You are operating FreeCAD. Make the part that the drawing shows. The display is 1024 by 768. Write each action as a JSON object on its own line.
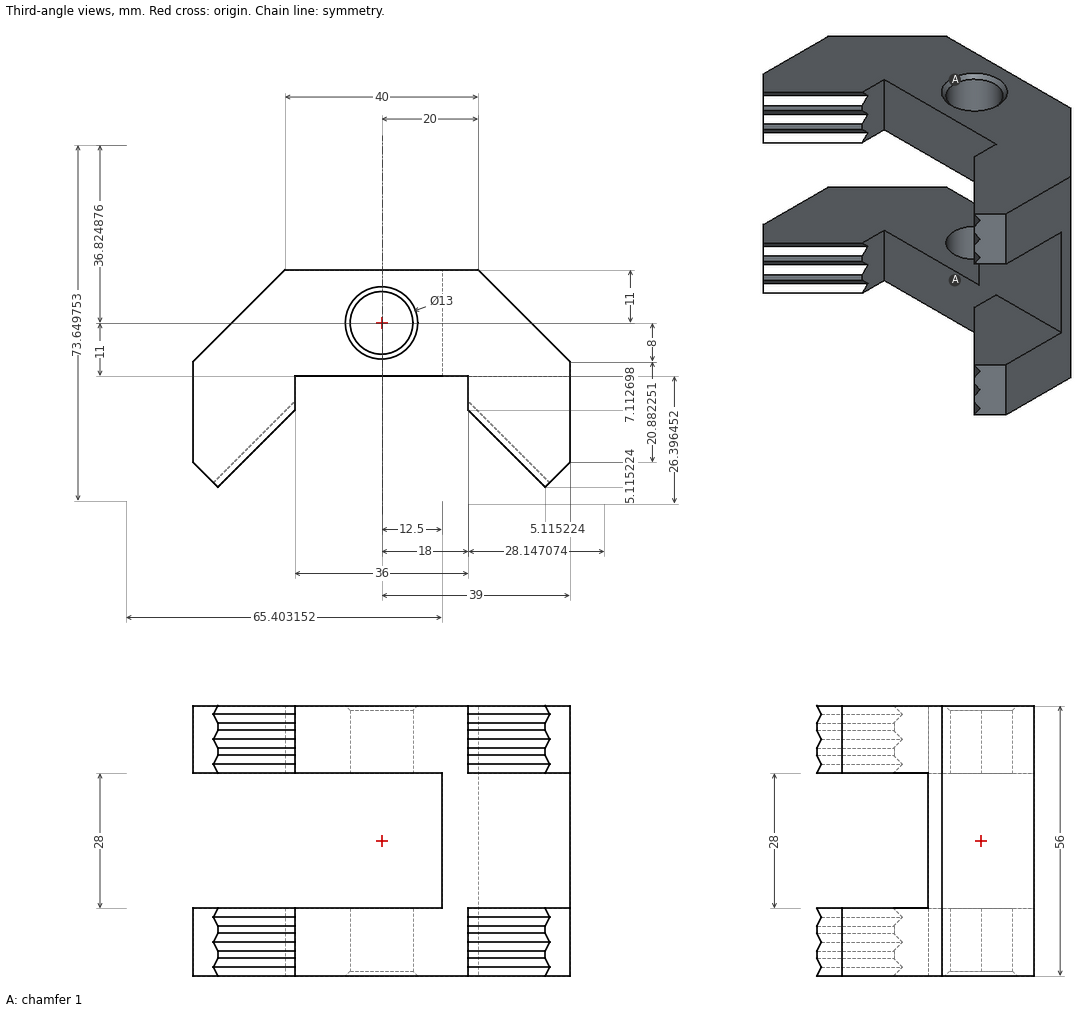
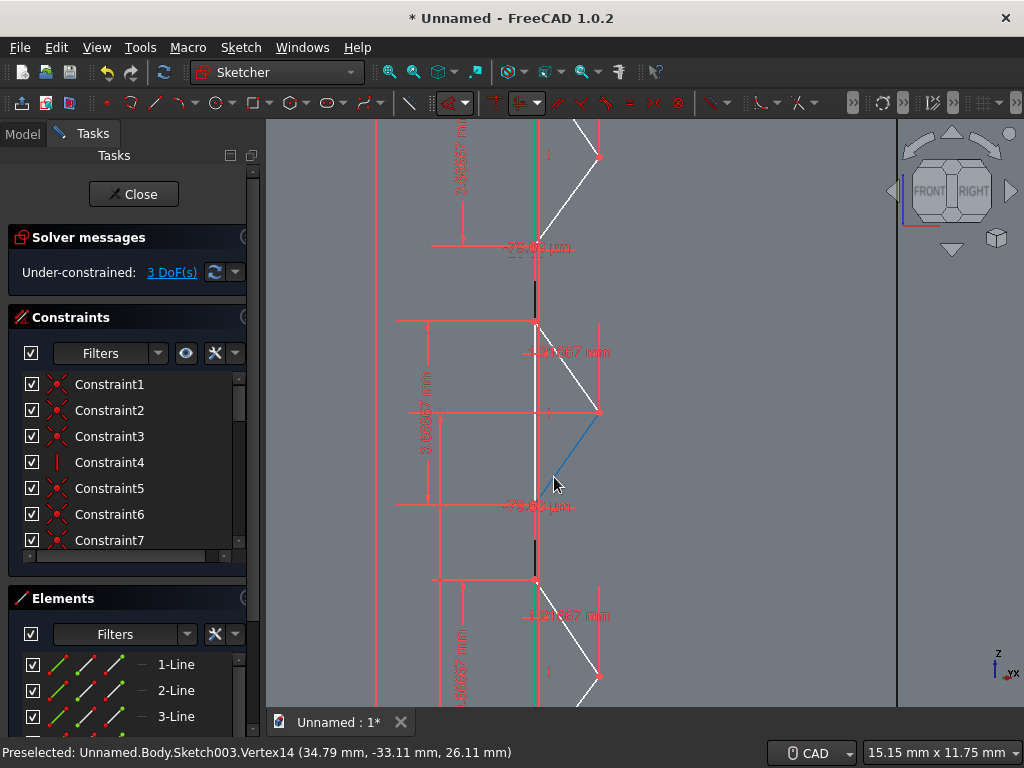
{"action": "left_click", "coordinate": [554, 477]}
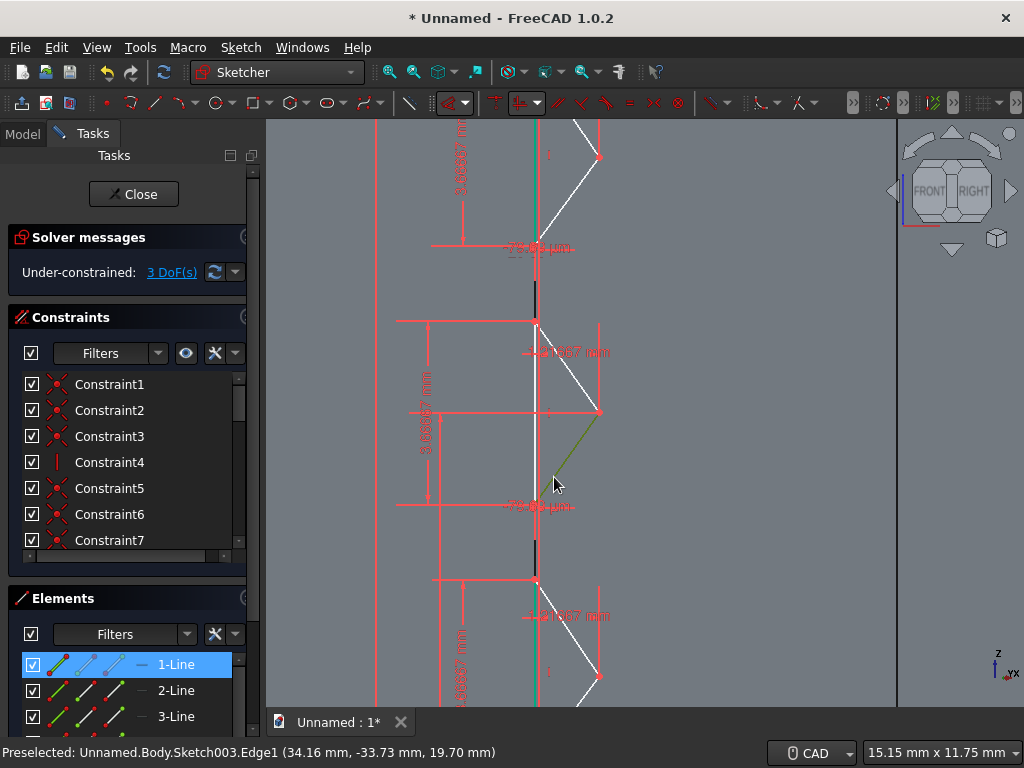
{"action": "key", "text": "i"}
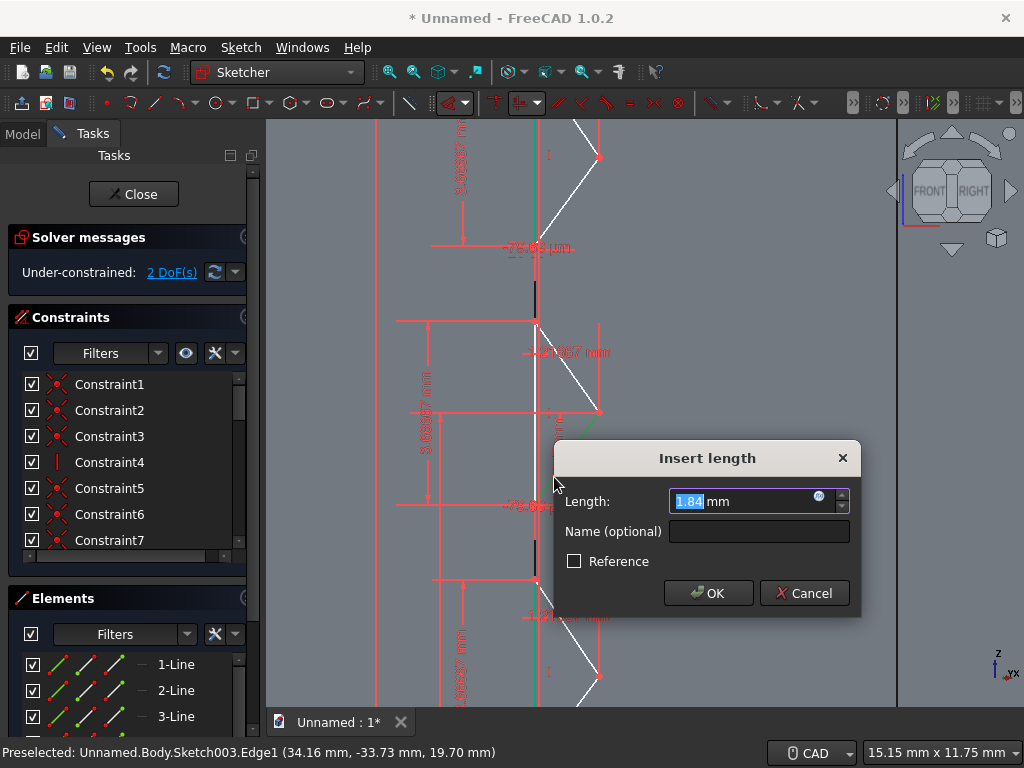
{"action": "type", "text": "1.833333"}
{"action": "key", "text": "Return"}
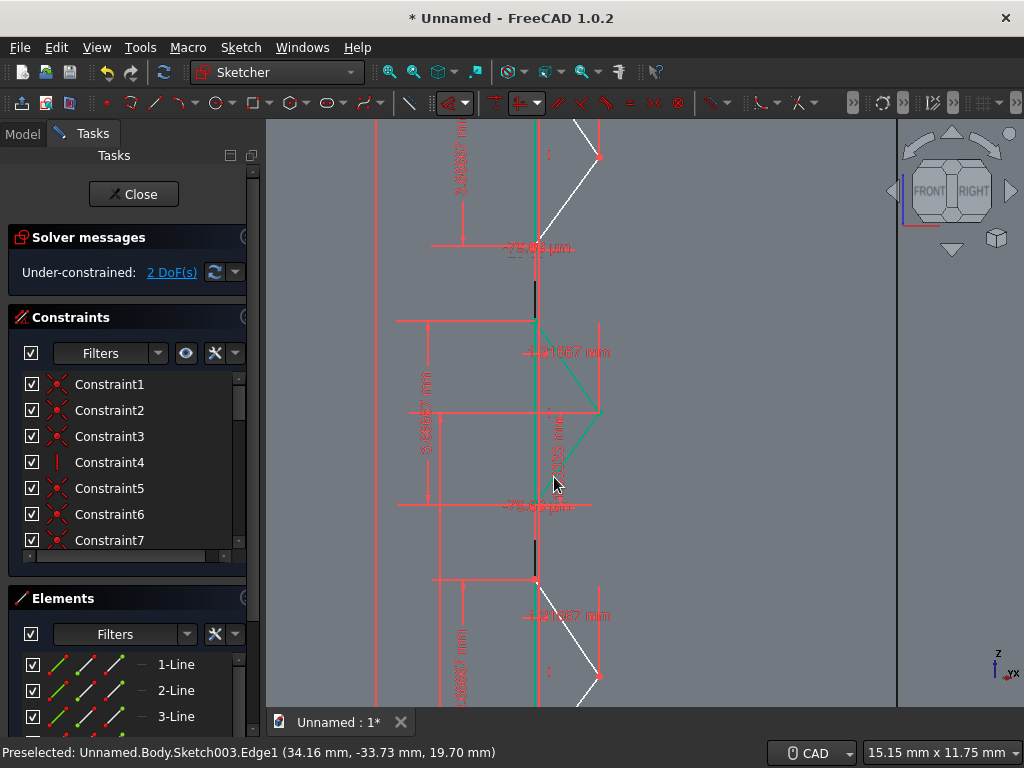
{"action": "scroll", "coordinate": [580, 298], "scroll_direction": "down", "scroll_amount": 7}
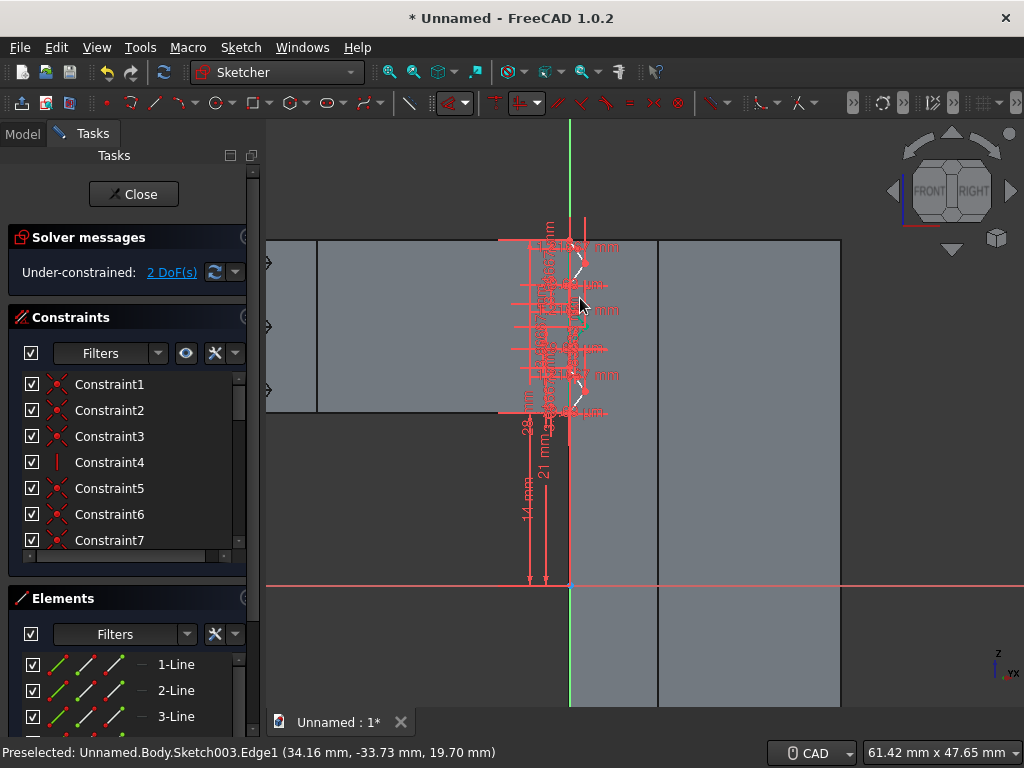
{"action": "scroll", "coordinate": [574, 406], "scroll_direction": "up", "scroll_amount": 7}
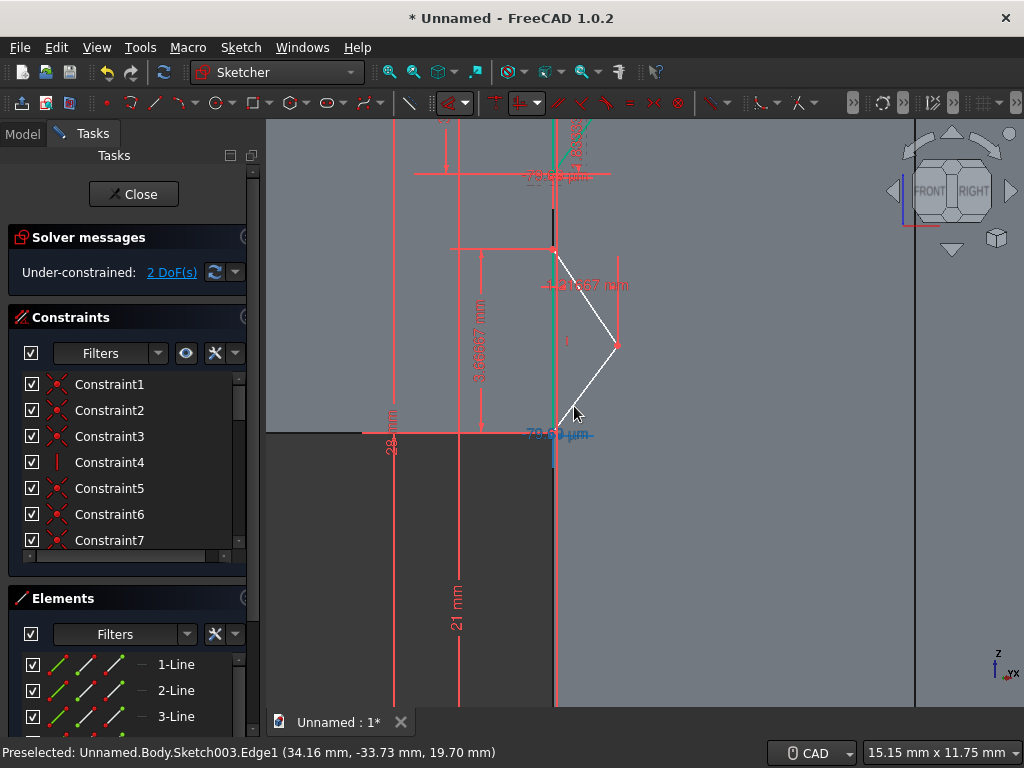
{"action": "left_click", "coordinate": [572, 407]}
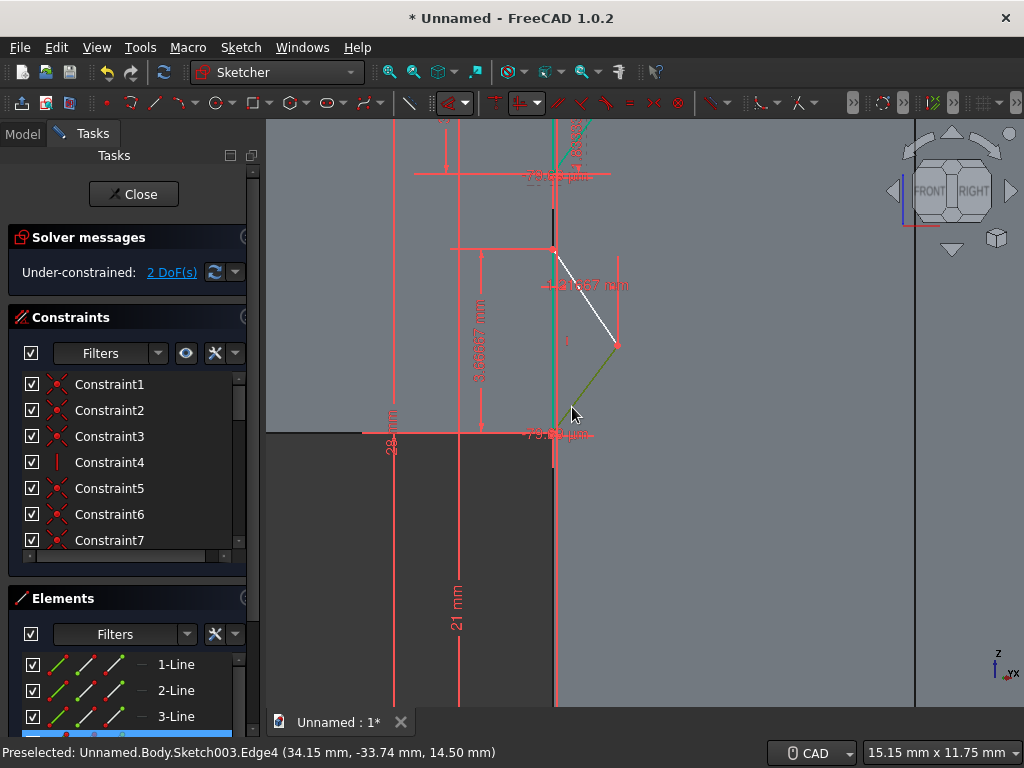
{"action": "left_click", "coordinate": [468, 104]}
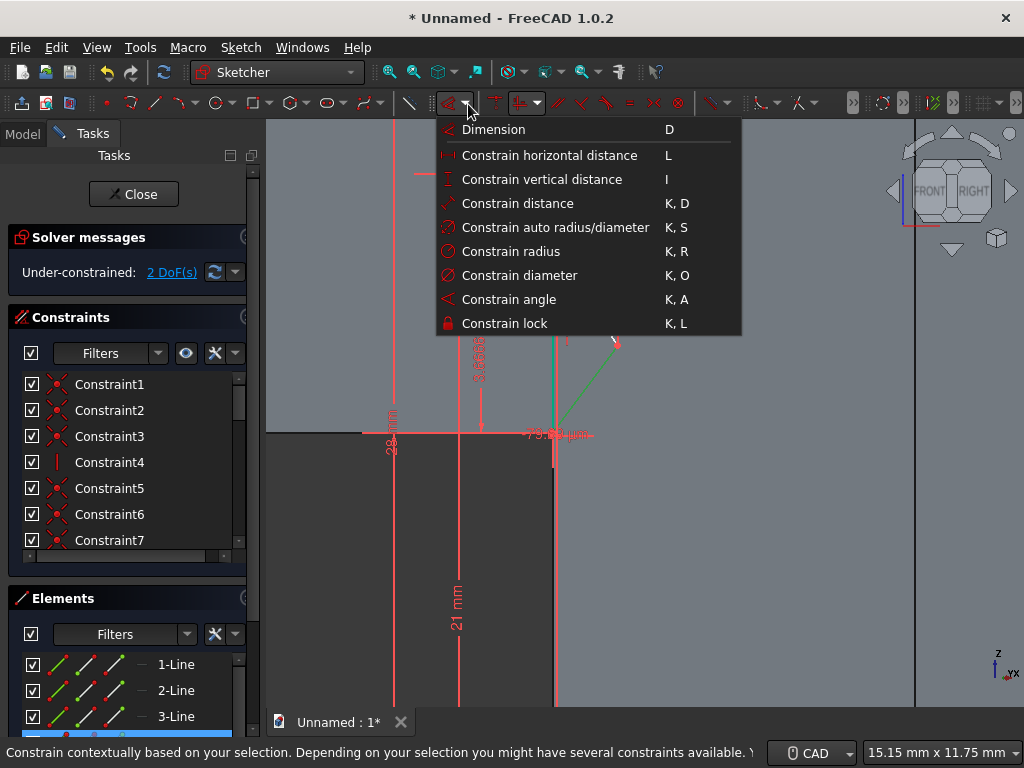
{"action": "left_click", "coordinate": [589, 179]}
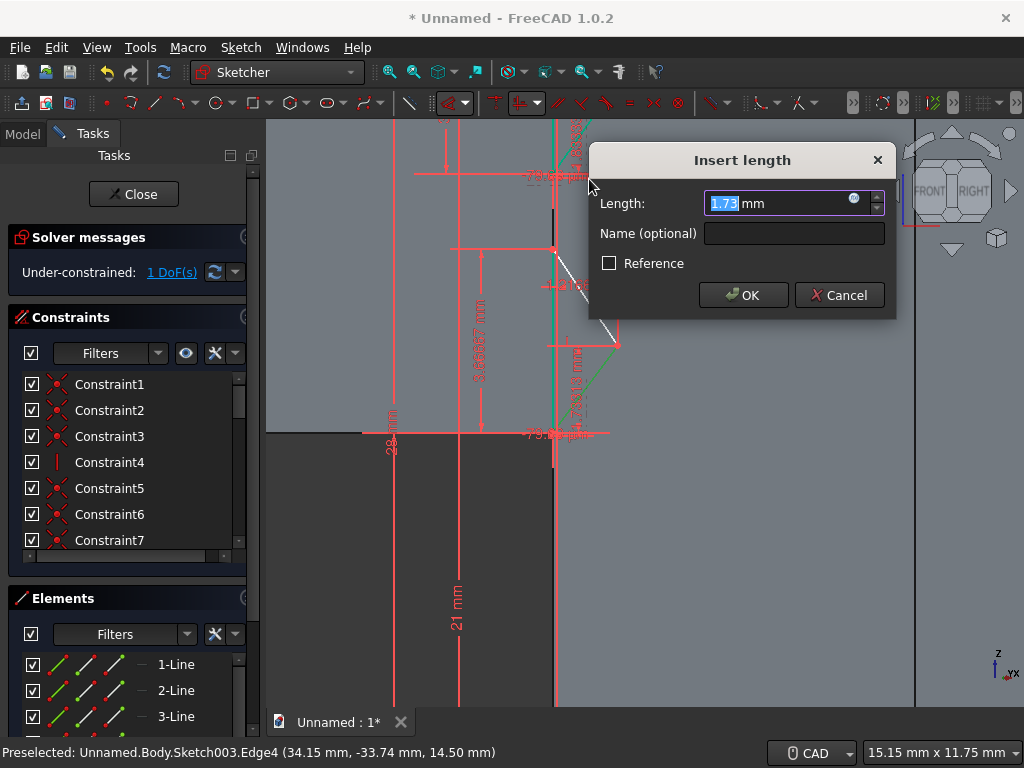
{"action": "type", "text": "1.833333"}
{"action": "key", "text": "Return"}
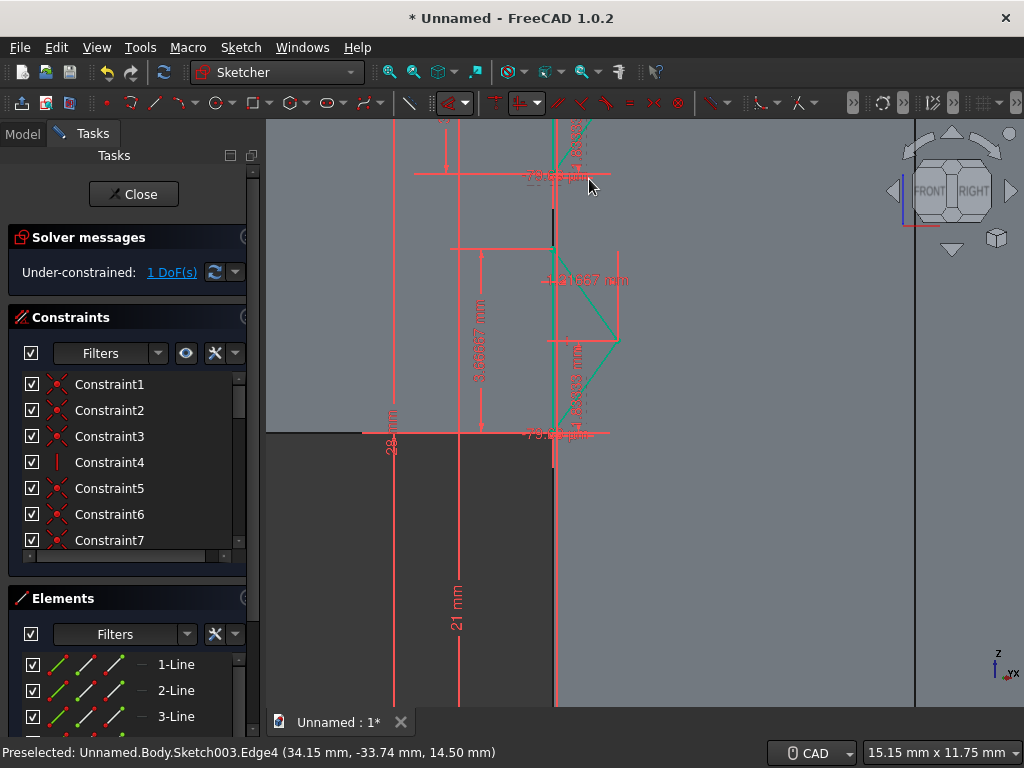
{"action": "scroll", "coordinate": [574, 407], "scroll_direction": "down", "scroll_amount": 7}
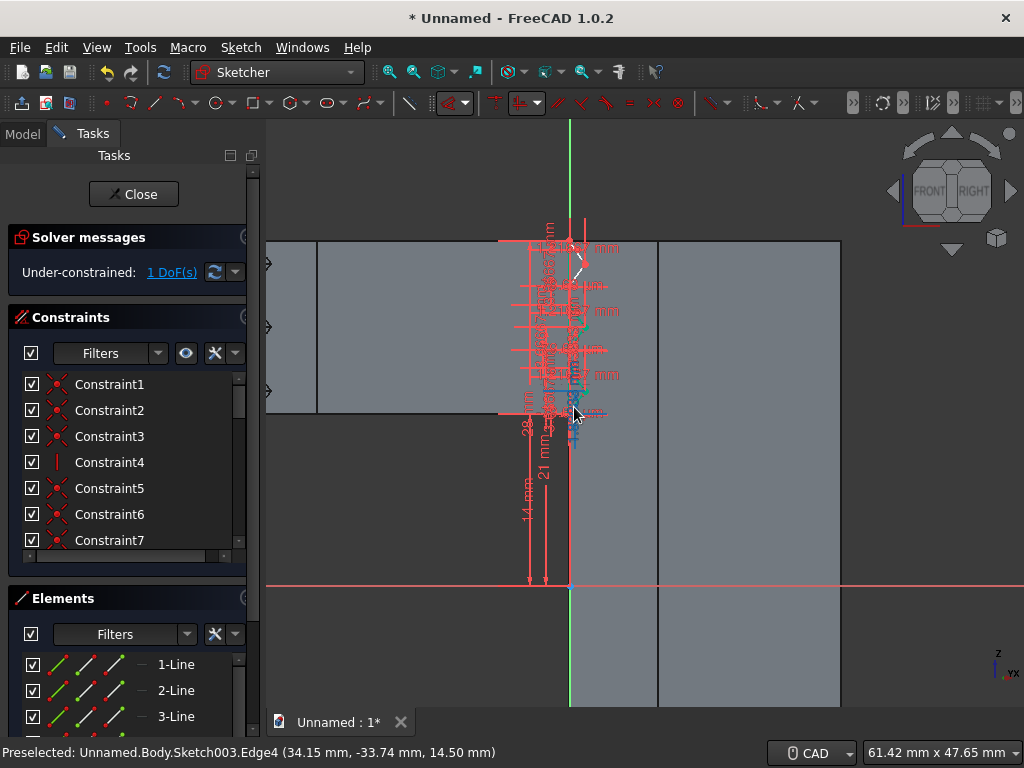
{"action": "scroll", "coordinate": [574, 280], "scroll_direction": "up", "scroll_amount": 7}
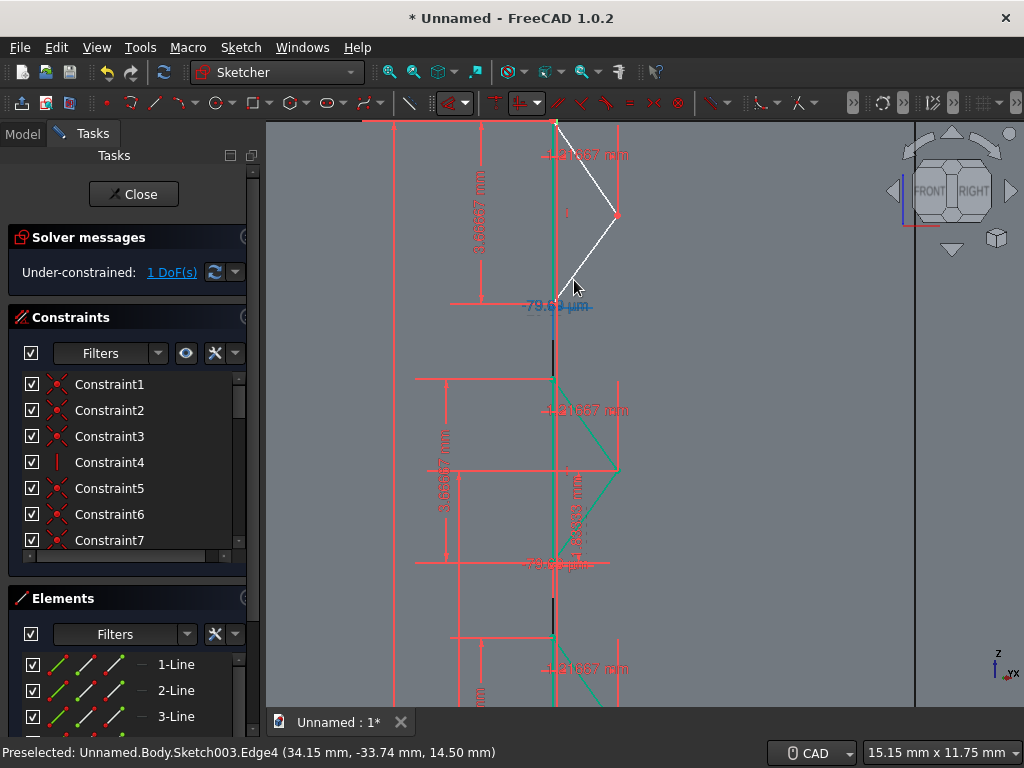
{"action": "left_click", "coordinate": [572, 277]}